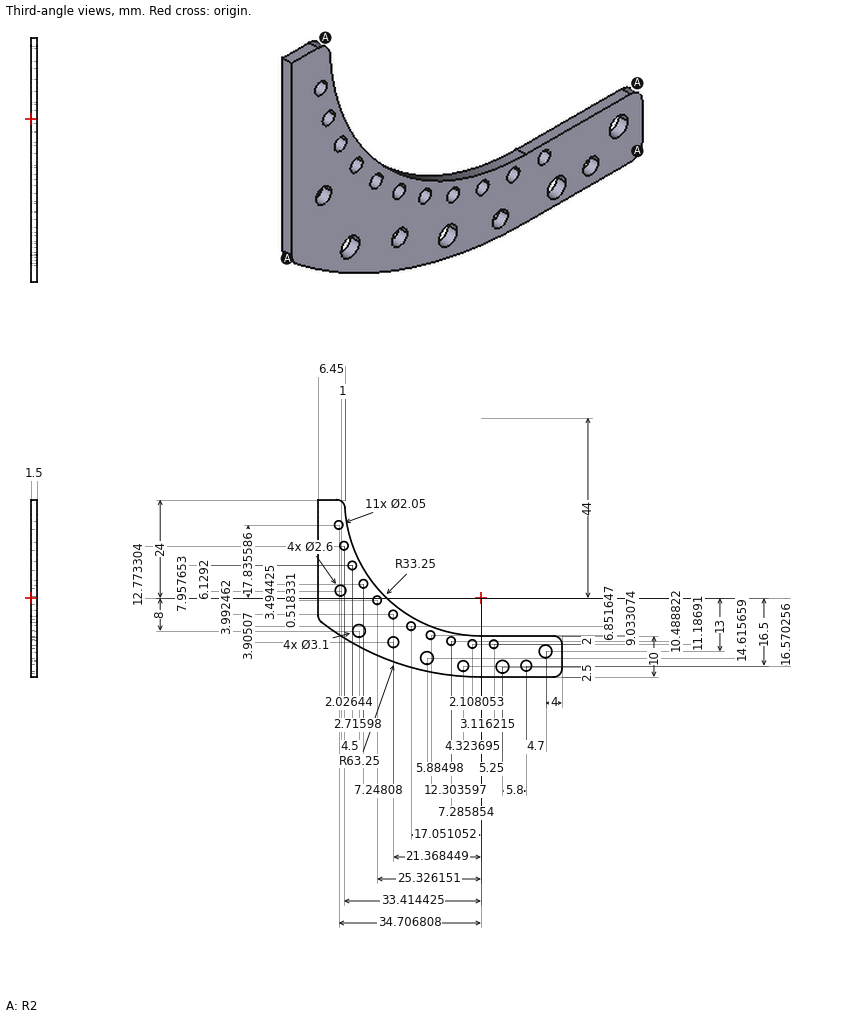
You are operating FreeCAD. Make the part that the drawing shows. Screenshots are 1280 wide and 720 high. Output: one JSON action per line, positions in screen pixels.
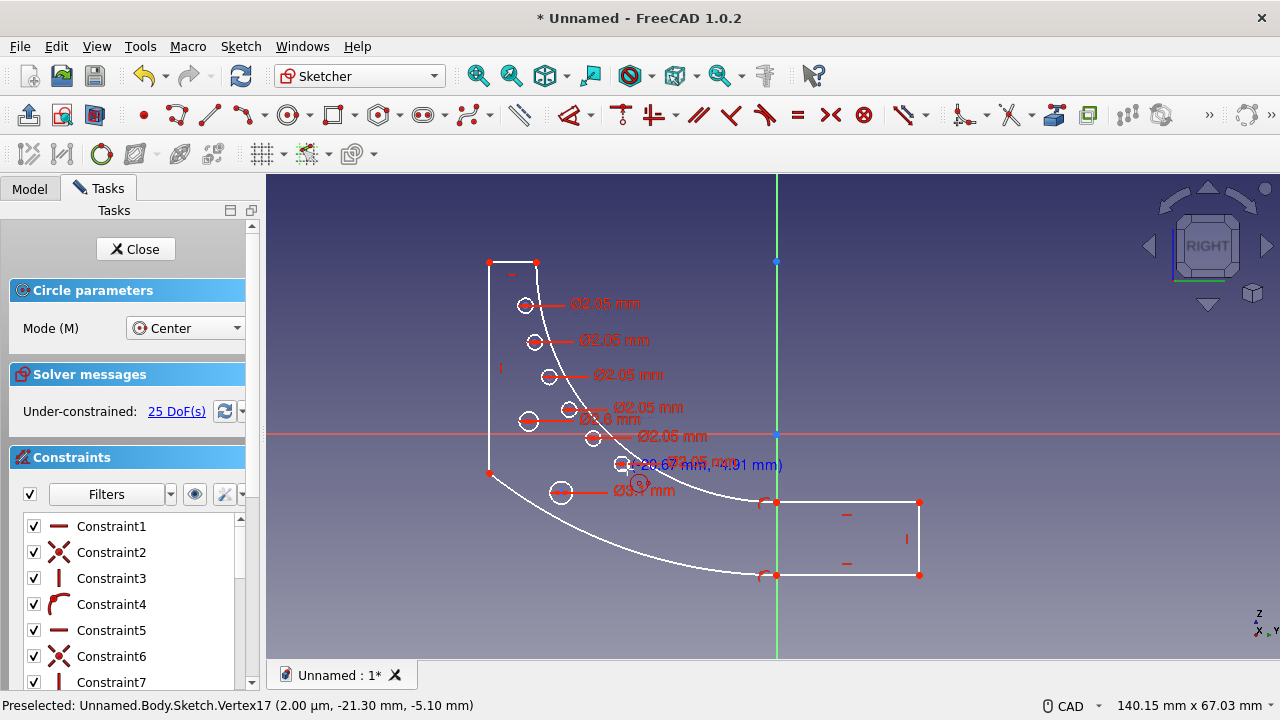
{"action": "scroll", "coordinate": [653, 484], "scroll_direction": "up", "scroll_amount": 6}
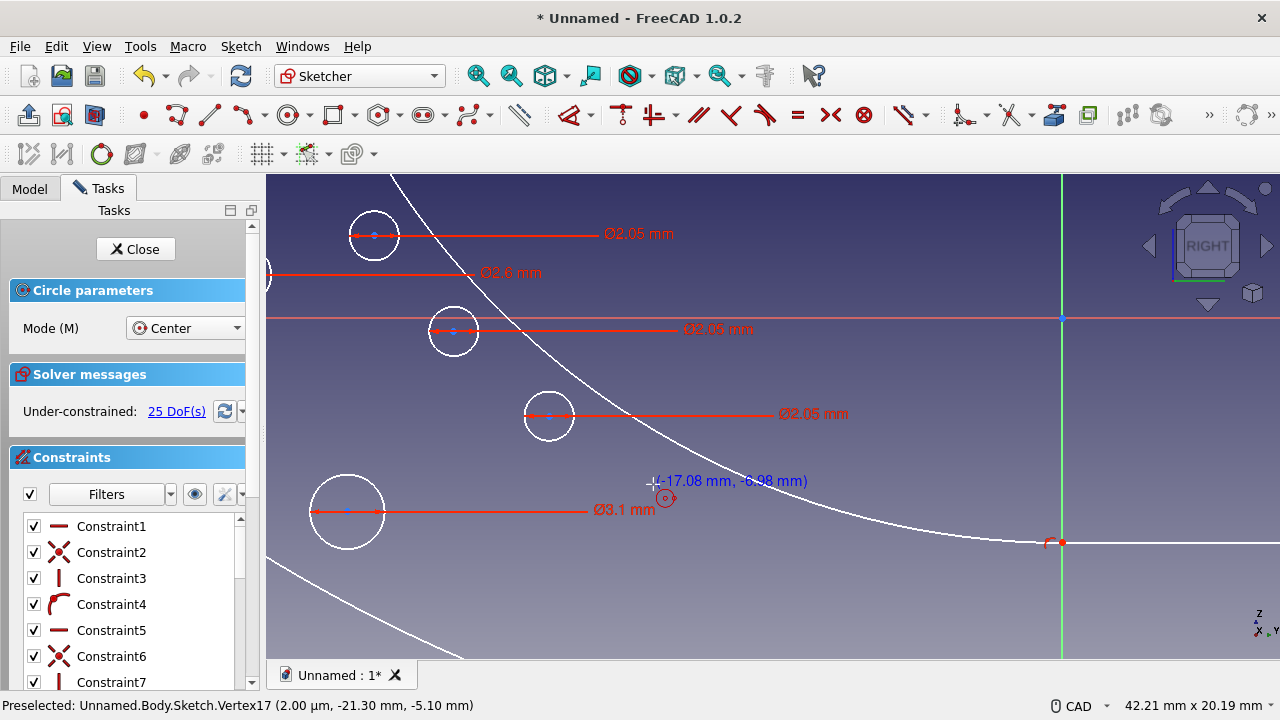
{"action": "left_click", "coordinate": [653, 483]}
{"action": "mouse_move", "coordinate": [670, 465]}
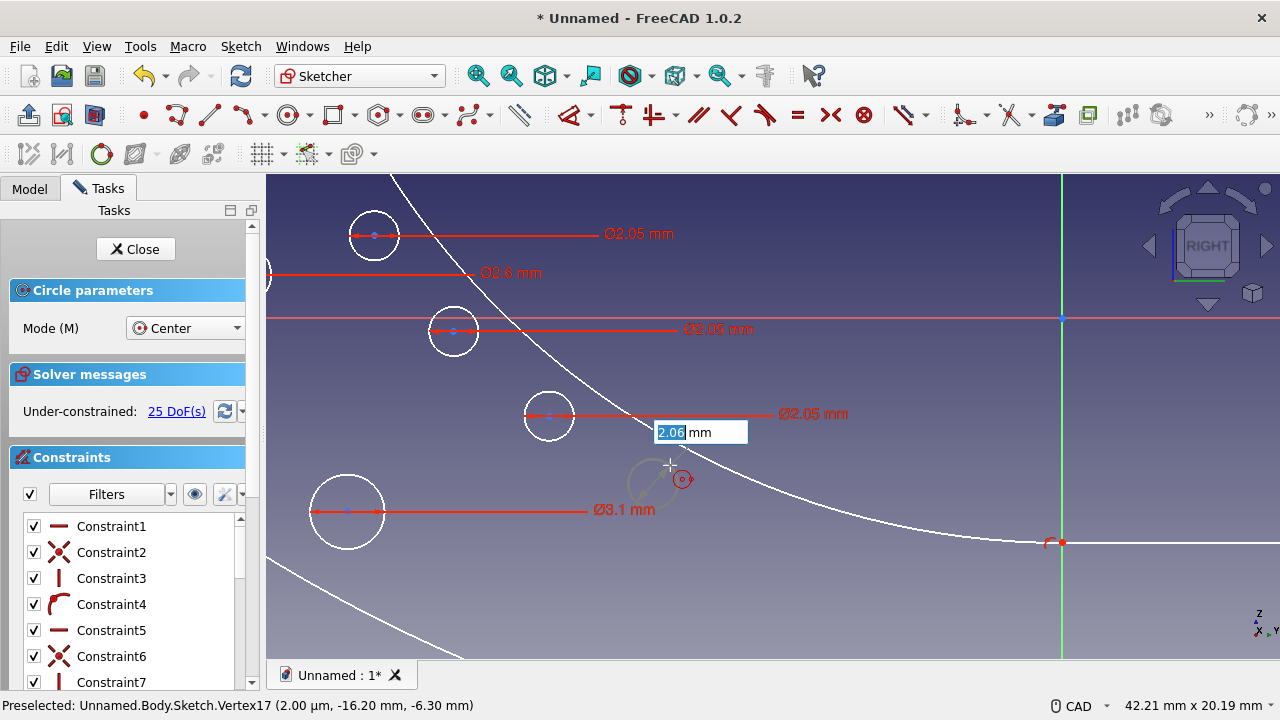
{"action": "type", "text": "2.05"}
{"action": "key", "text": "Return"}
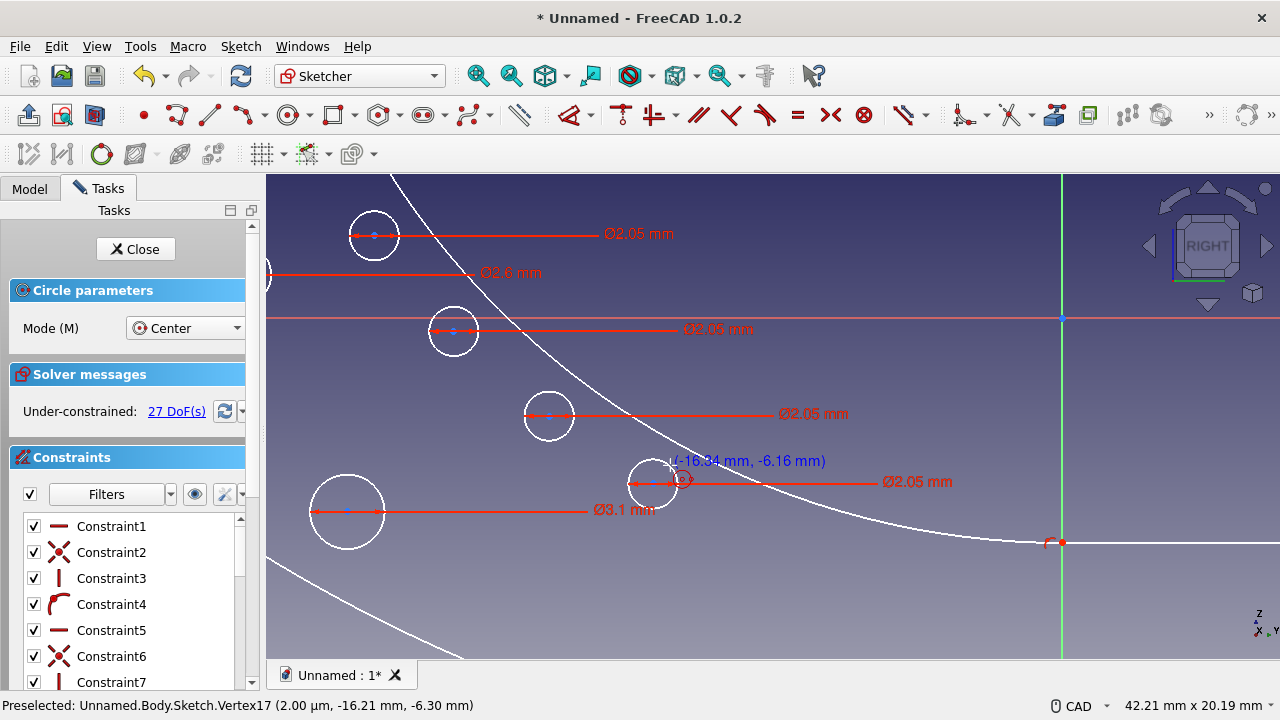
{"action": "left_click", "coordinate": [549, 576]}
{"action": "mouse_move", "coordinate": [571, 554]}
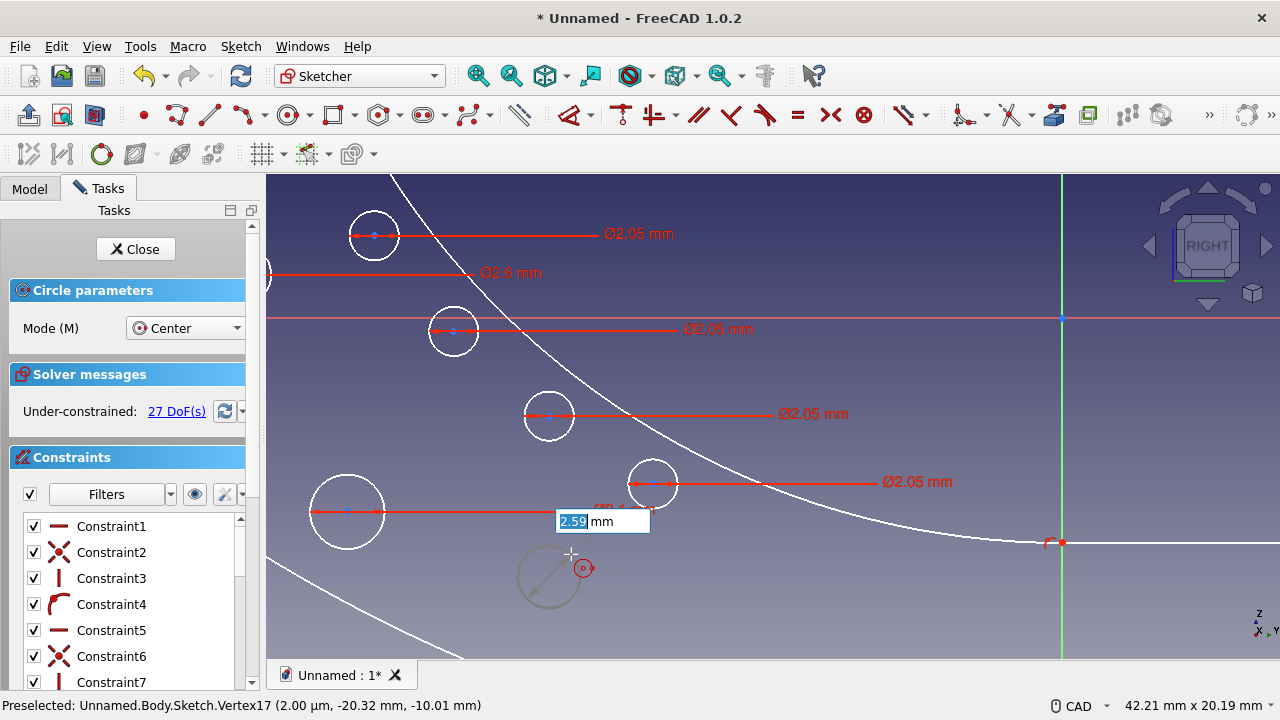
{"action": "type", "text": "2.6"}
{"action": "key", "text": "Return"}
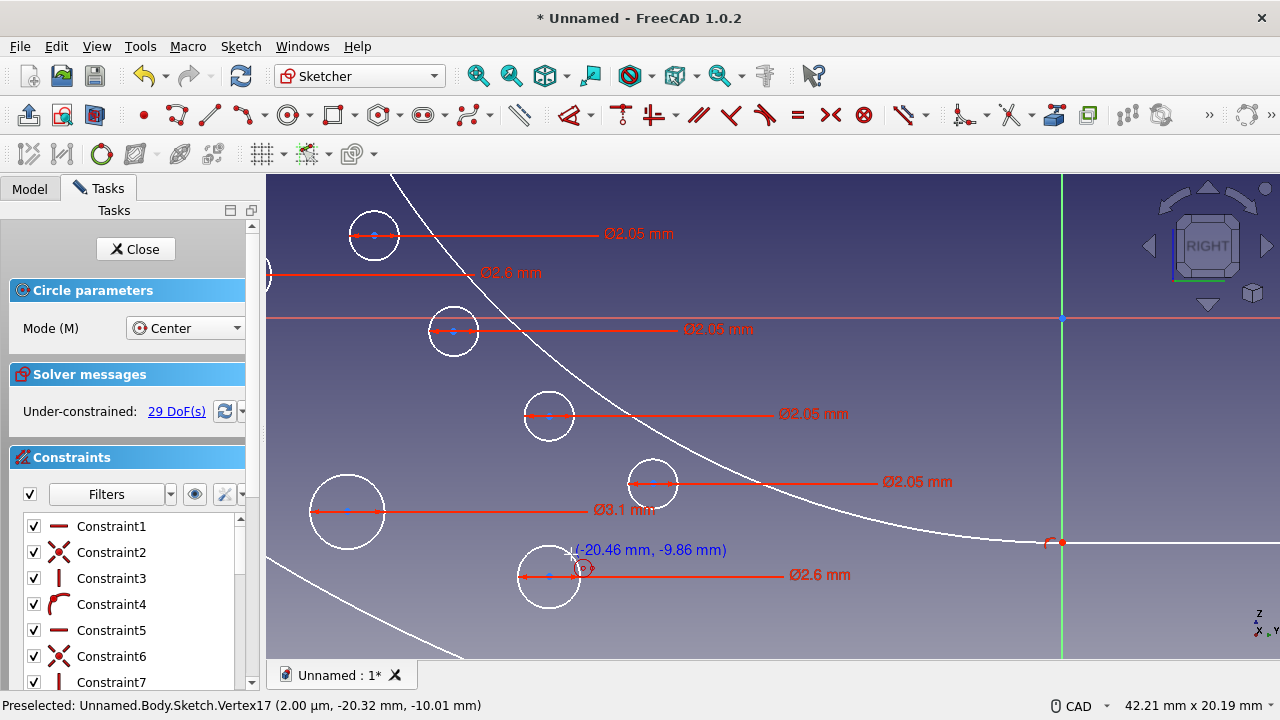
{"action": "left_click", "coordinate": [767, 535]}
{"action": "mouse_move", "coordinate": [784, 518]}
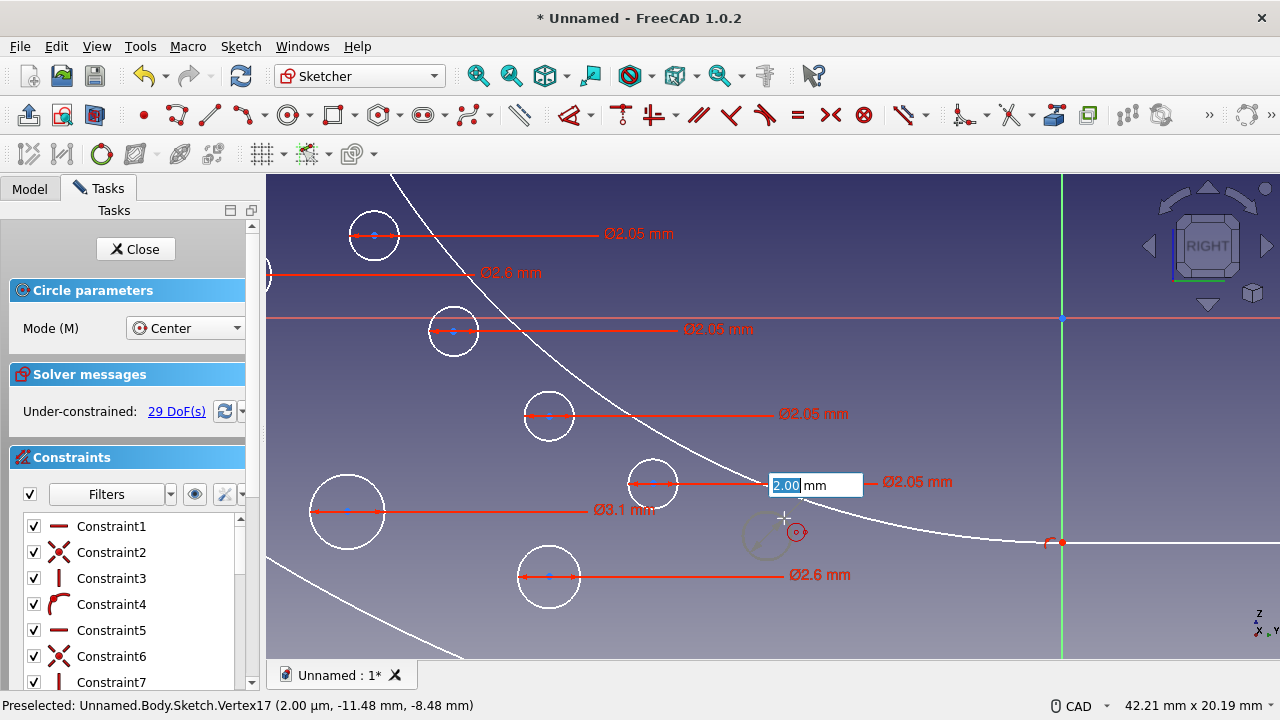
{"action": "type", "text": "2.05"}
{"action": "key", "text": "Return"}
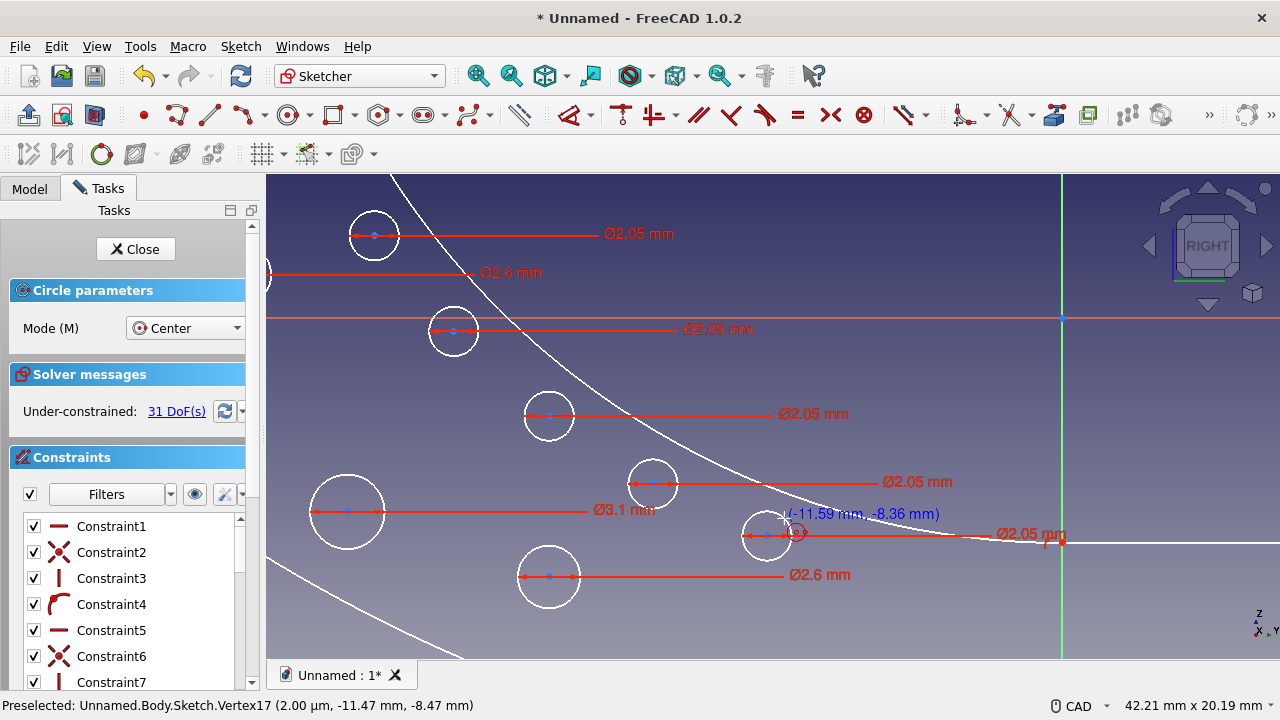
{"action": "scroll", "coordinate": [654, 484], "scroll_direction": "down", "scroll_amount": 6}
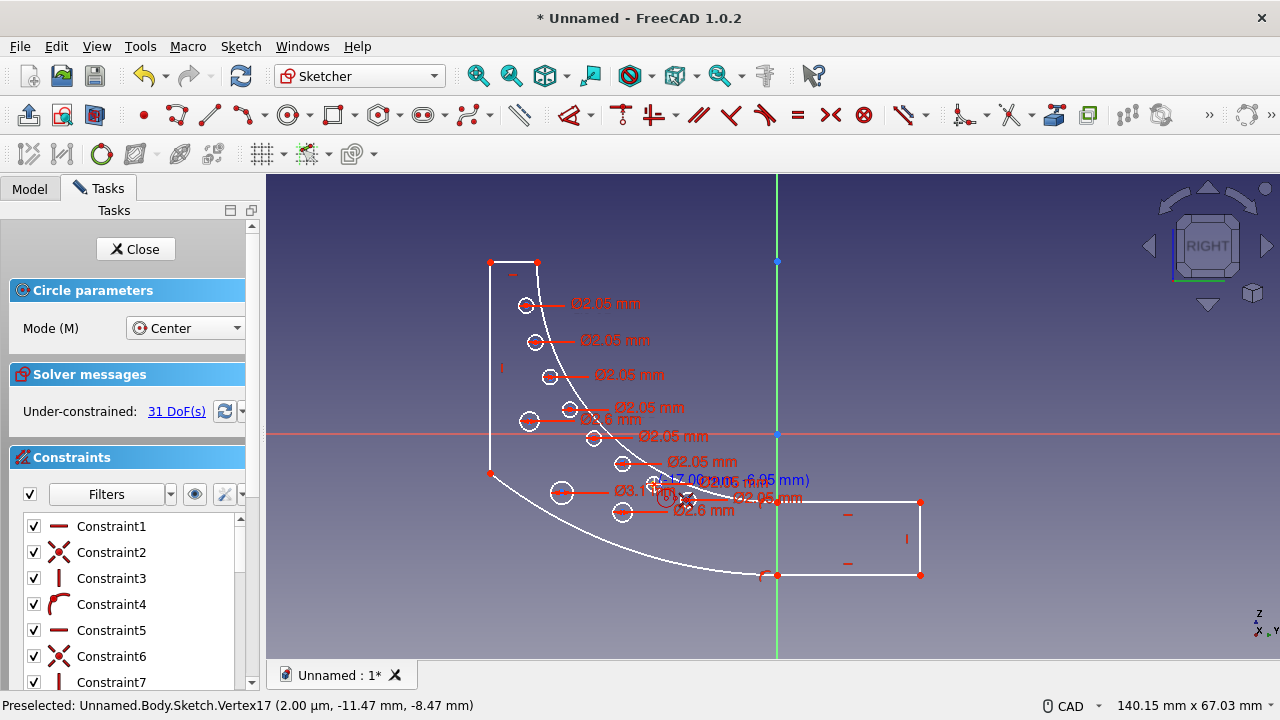
{"action": "scroll", "coordinate": [682, 540], "scroll_direction": "up", "scroll_amount": 4}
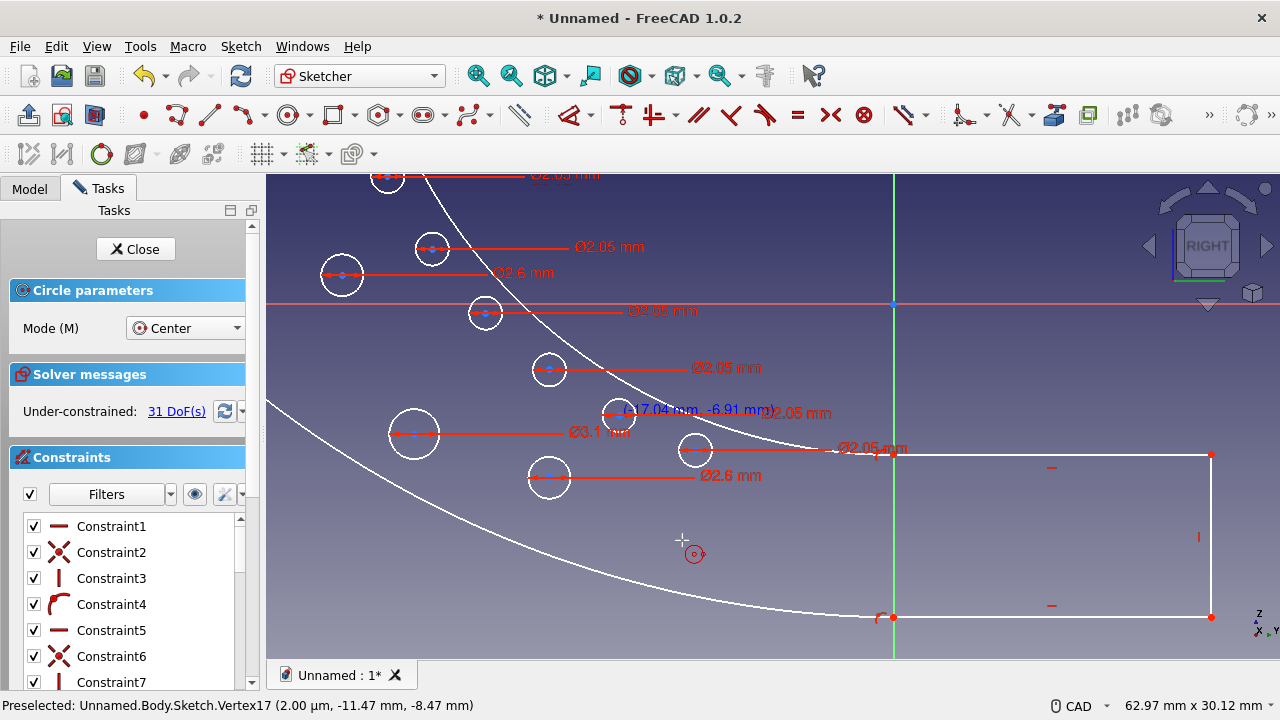
{"action": "left_click", "coordinate": [681, 540]}
{"action": "mouse_move", "coordinate": [699, 522]}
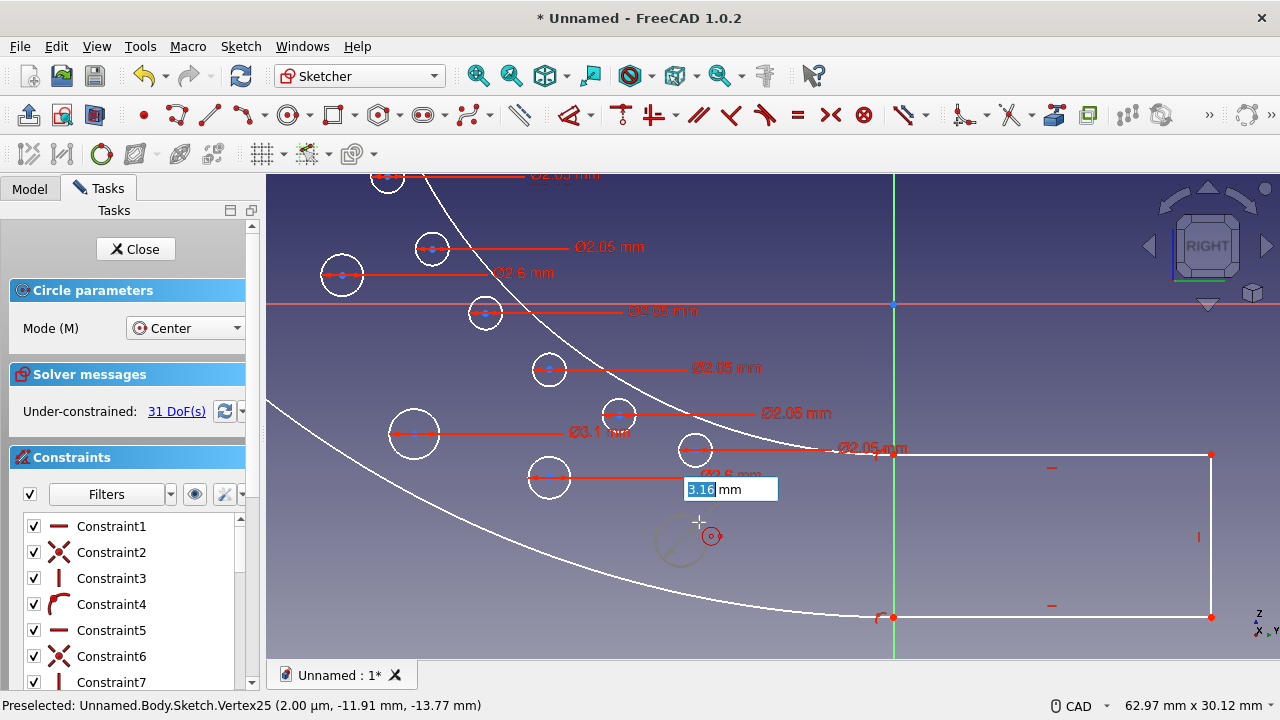
{"action": "type", "text": "3.1"}
{"action": "key", "text": "Return"}